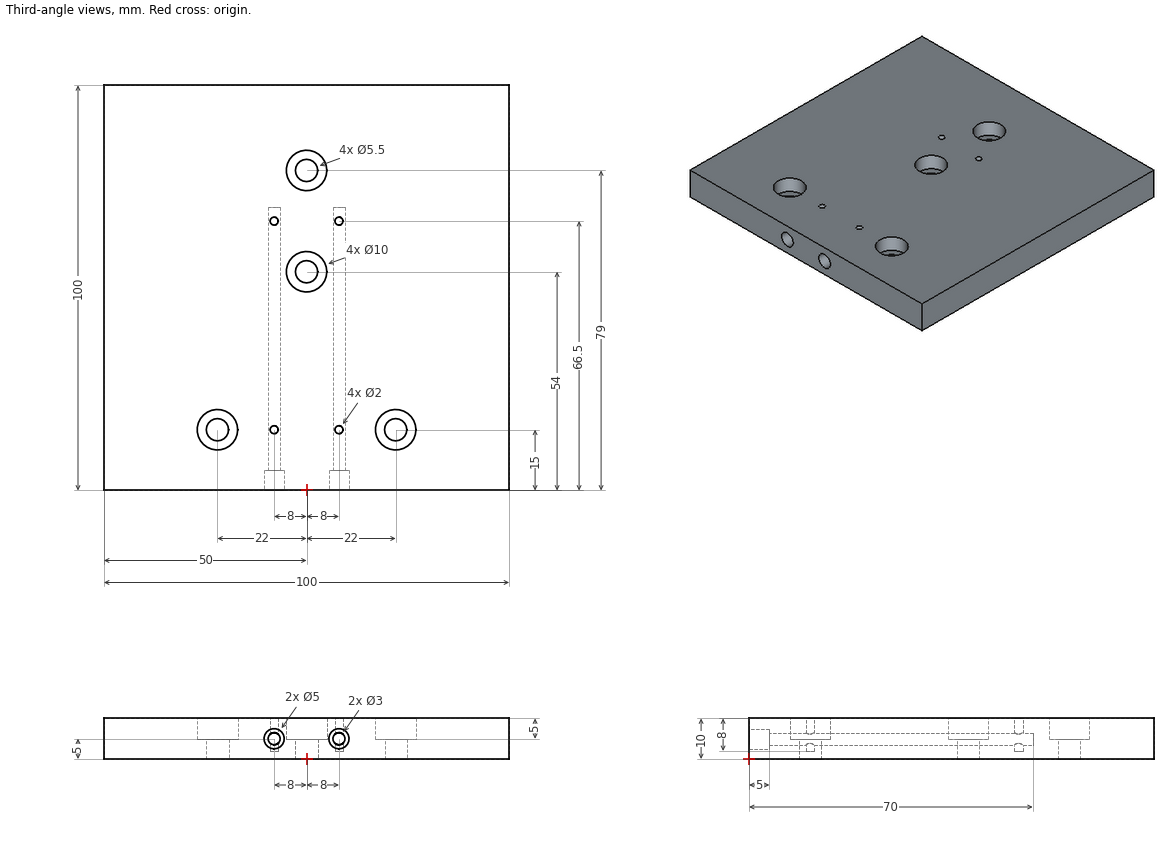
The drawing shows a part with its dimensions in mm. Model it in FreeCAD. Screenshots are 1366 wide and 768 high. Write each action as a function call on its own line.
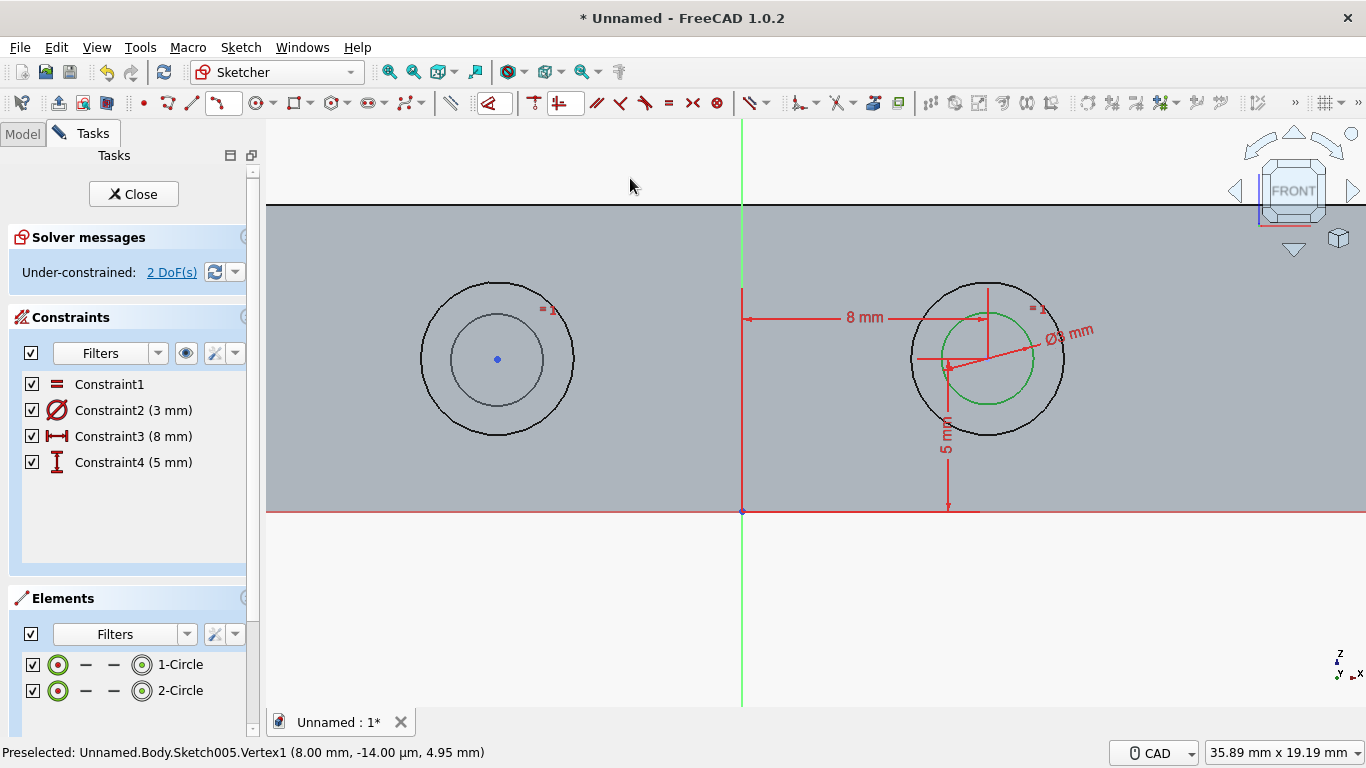
click(497, 360)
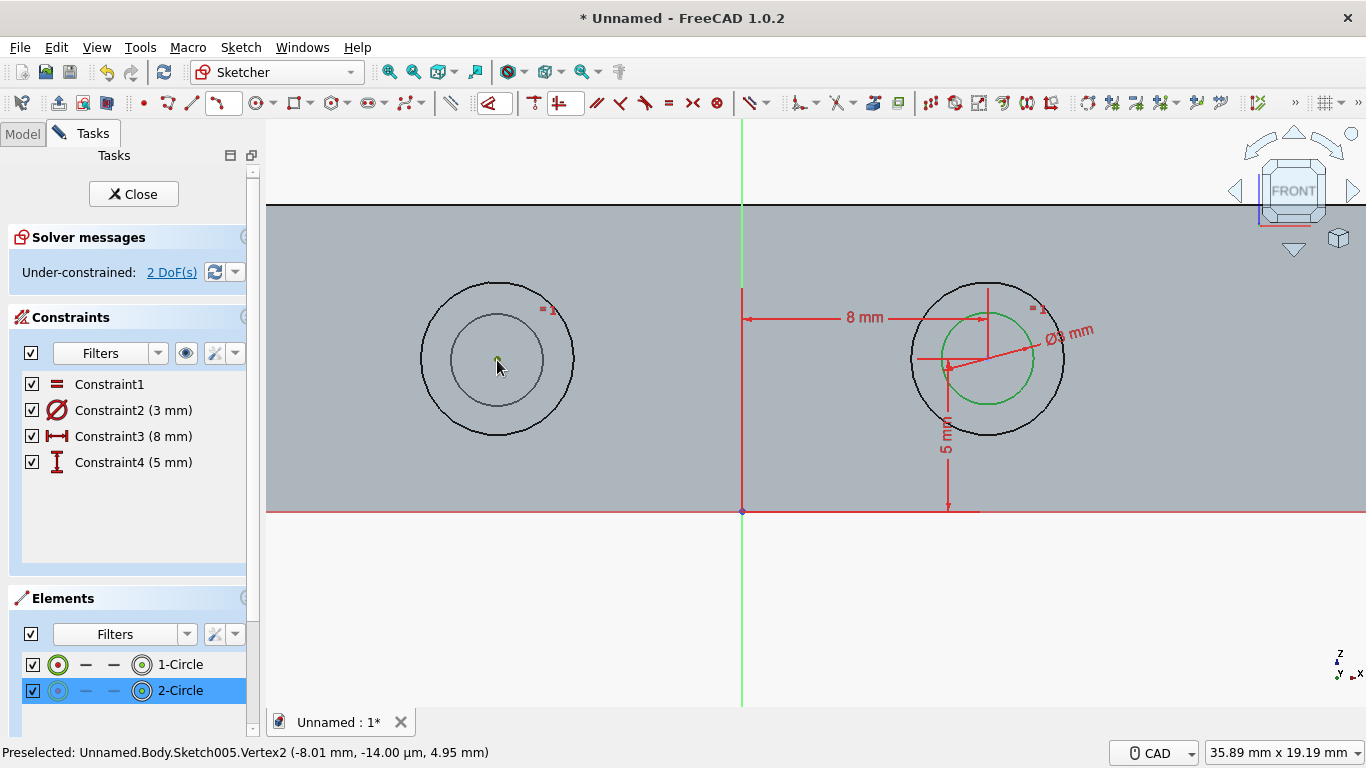
key(l)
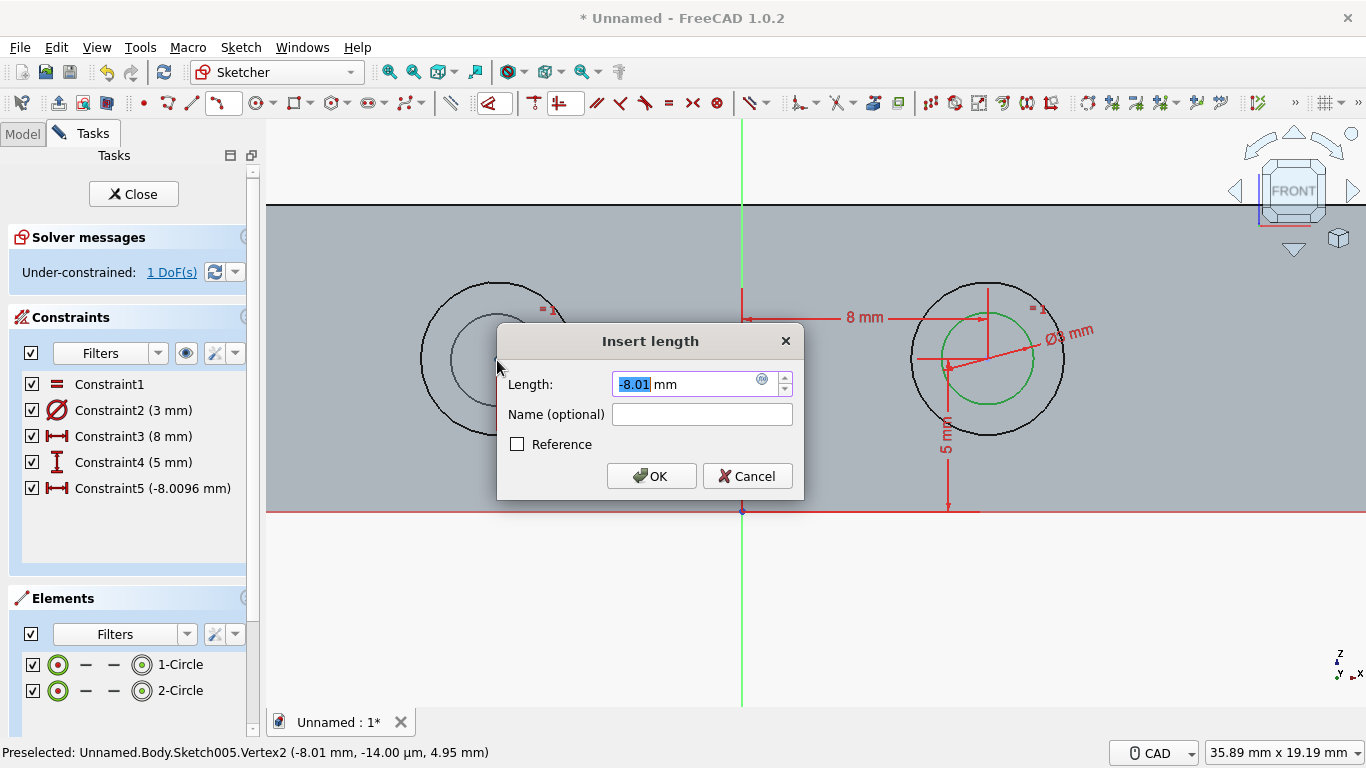
text(-8)
key(Return)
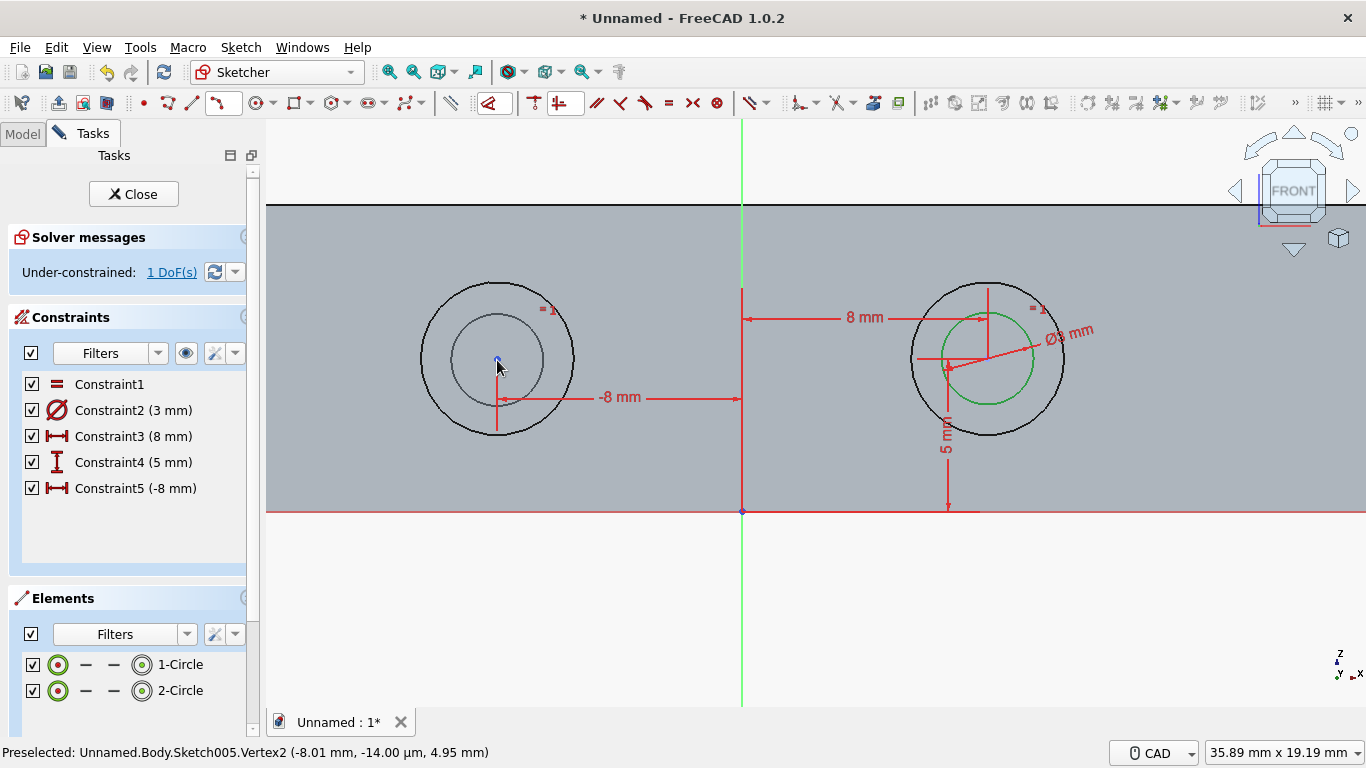
click(497, 360)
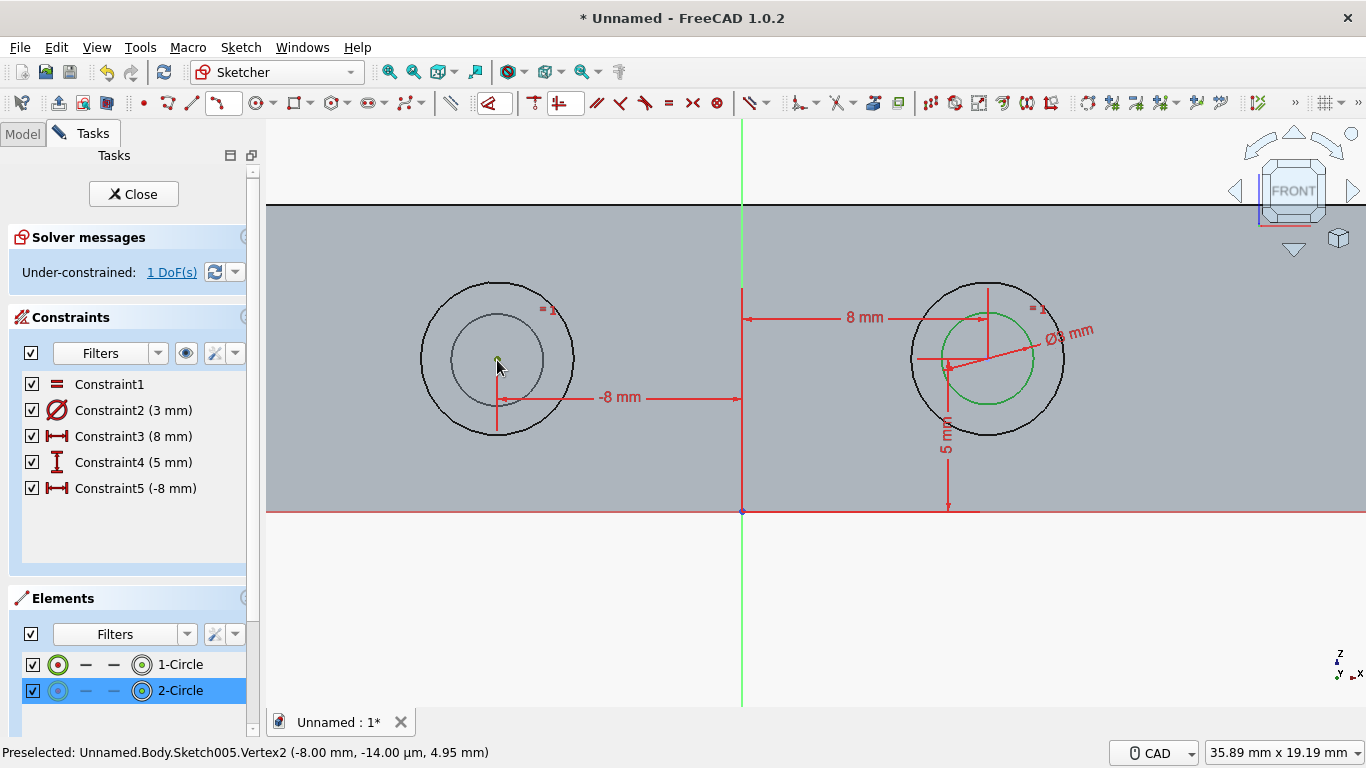
key(i)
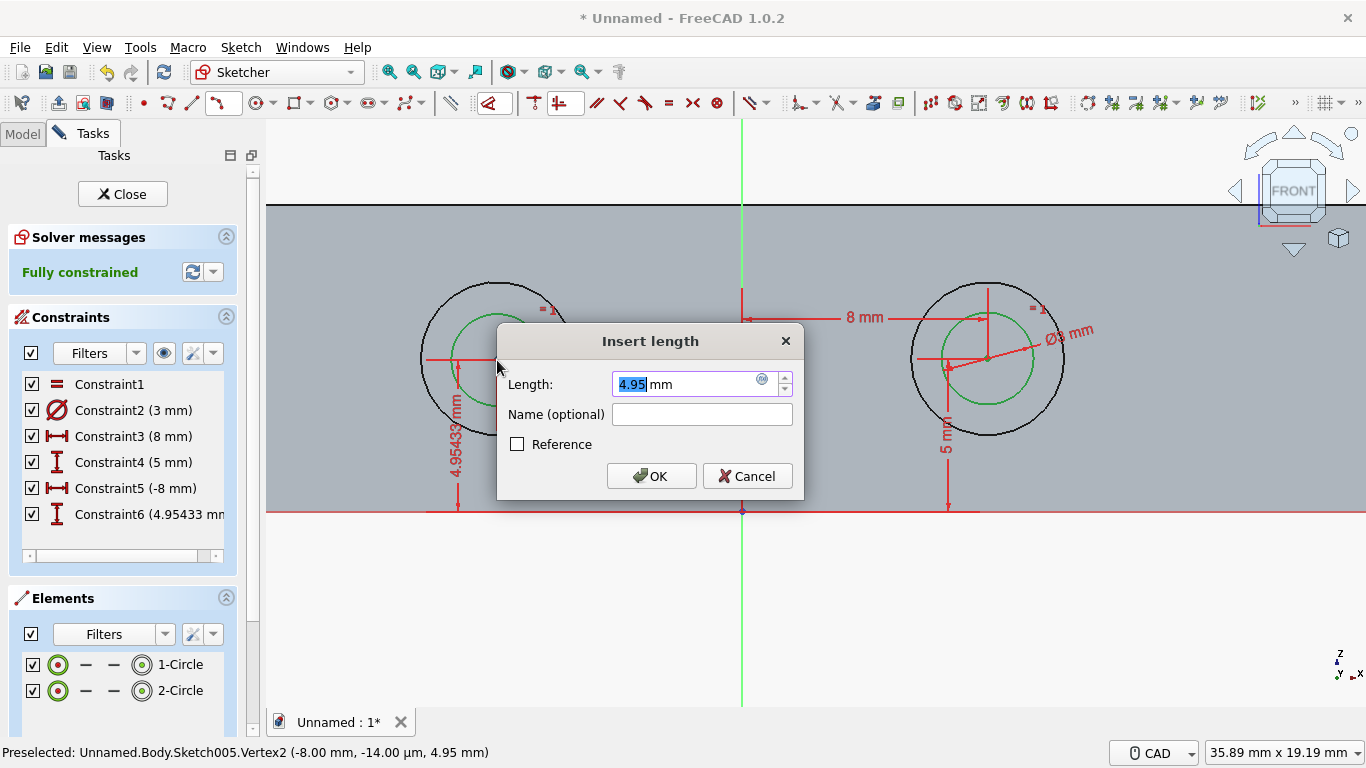
text(5)
key(Return)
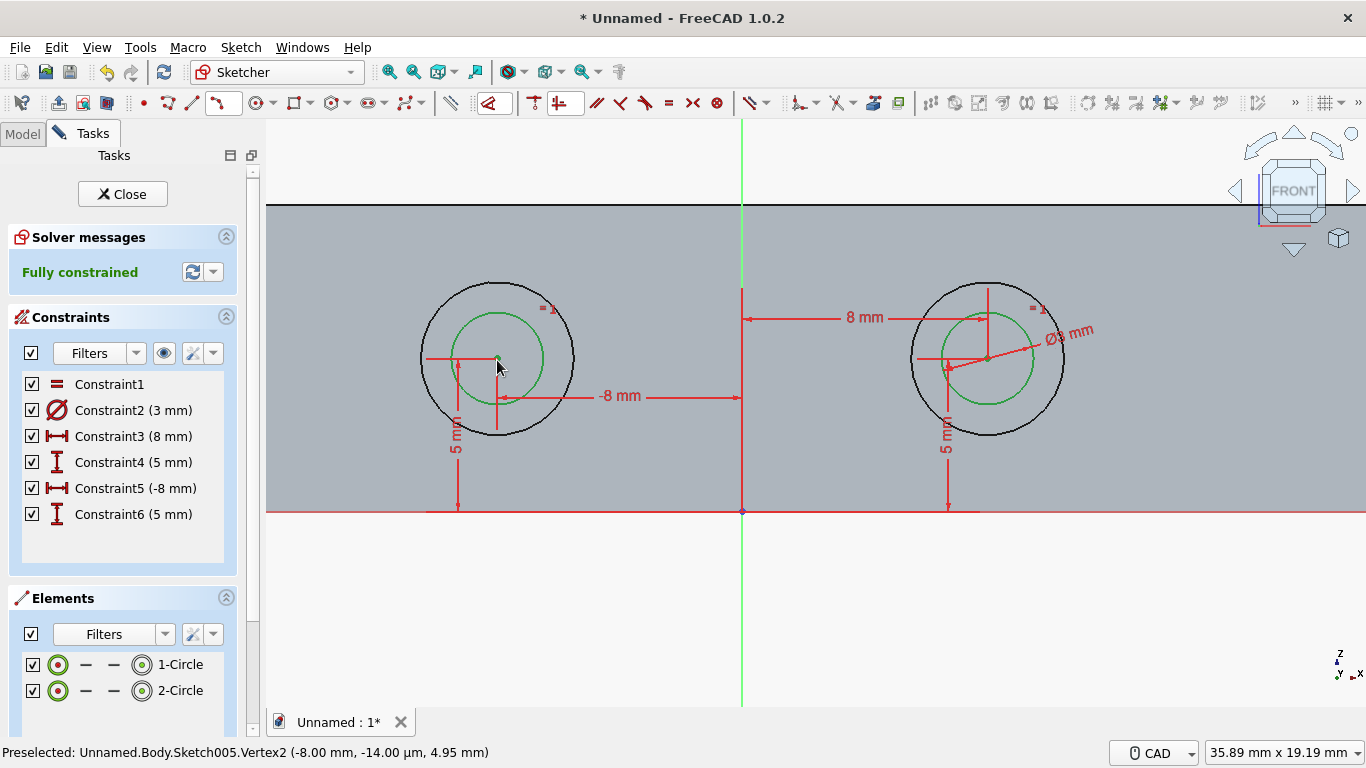
click(123, 194)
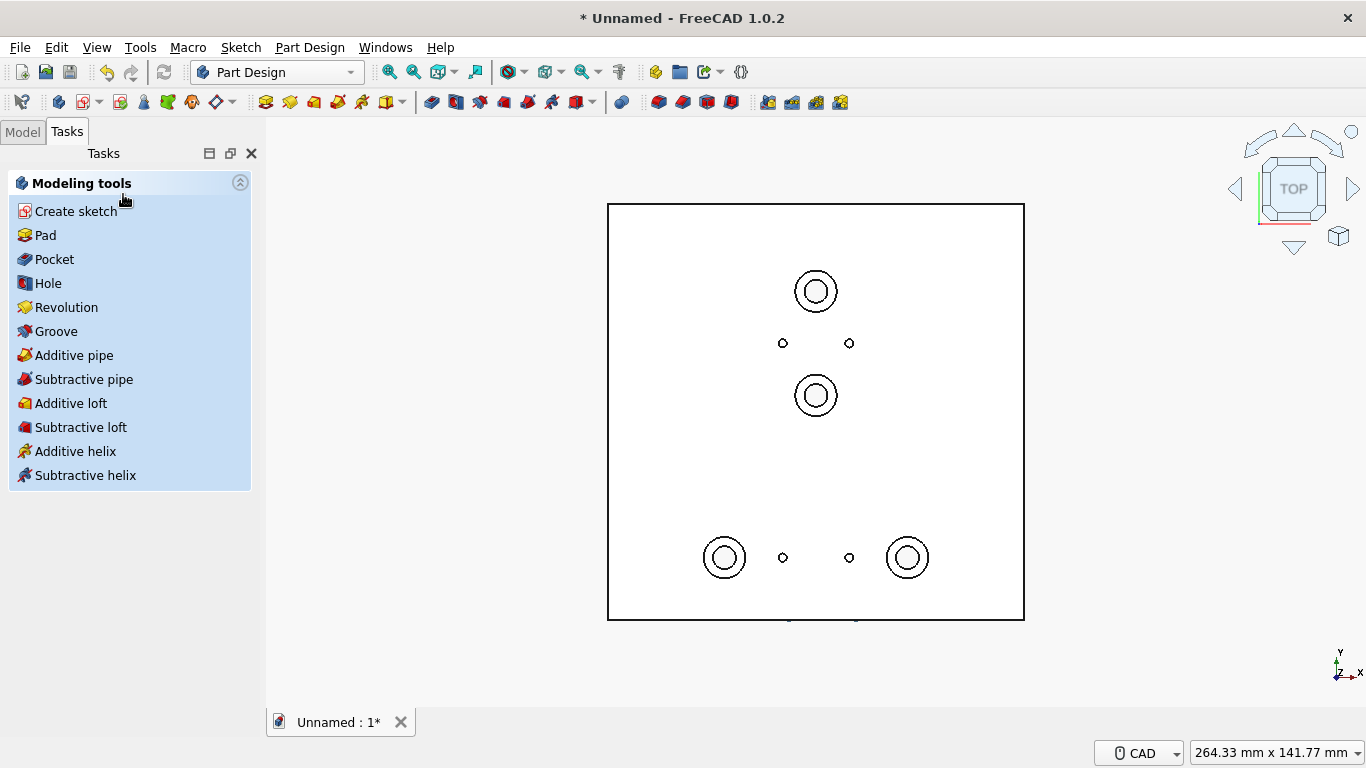
click(432, 102)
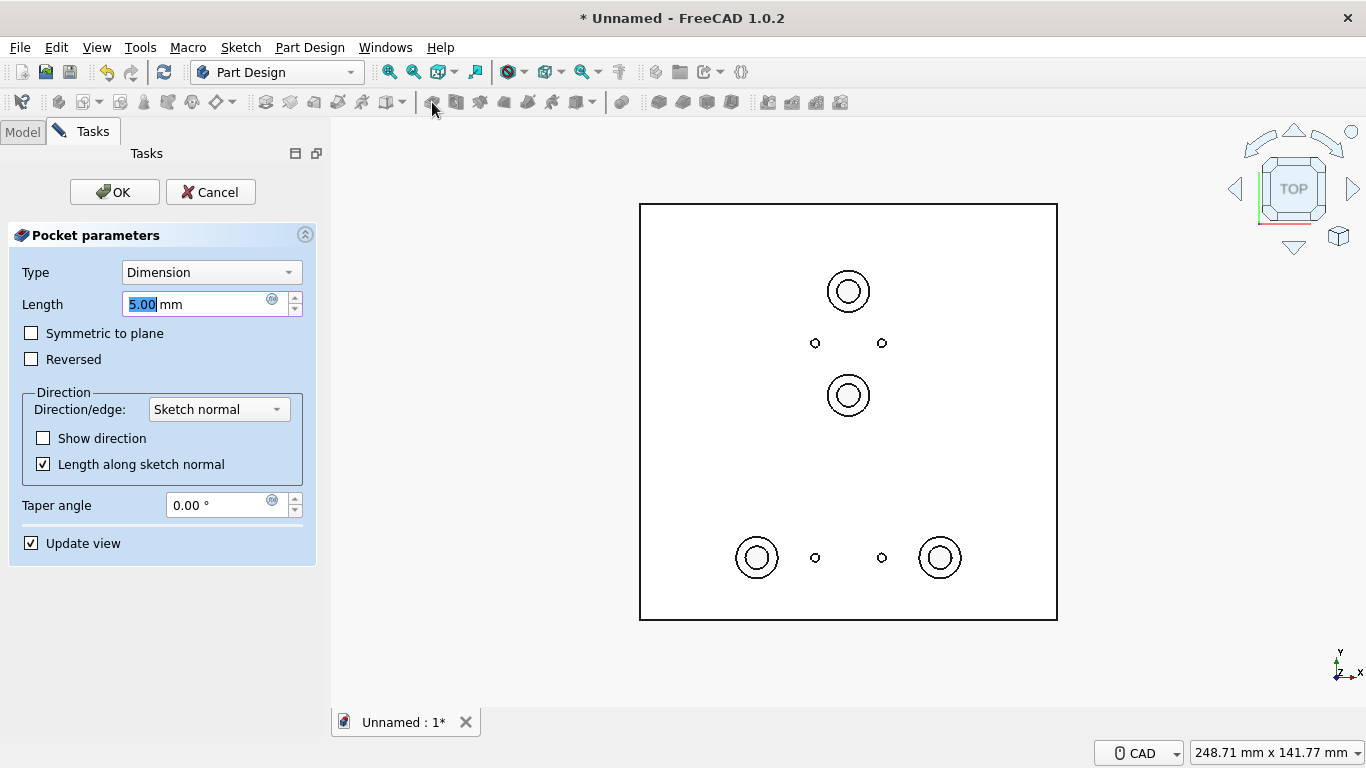
text(70)
key(Tab)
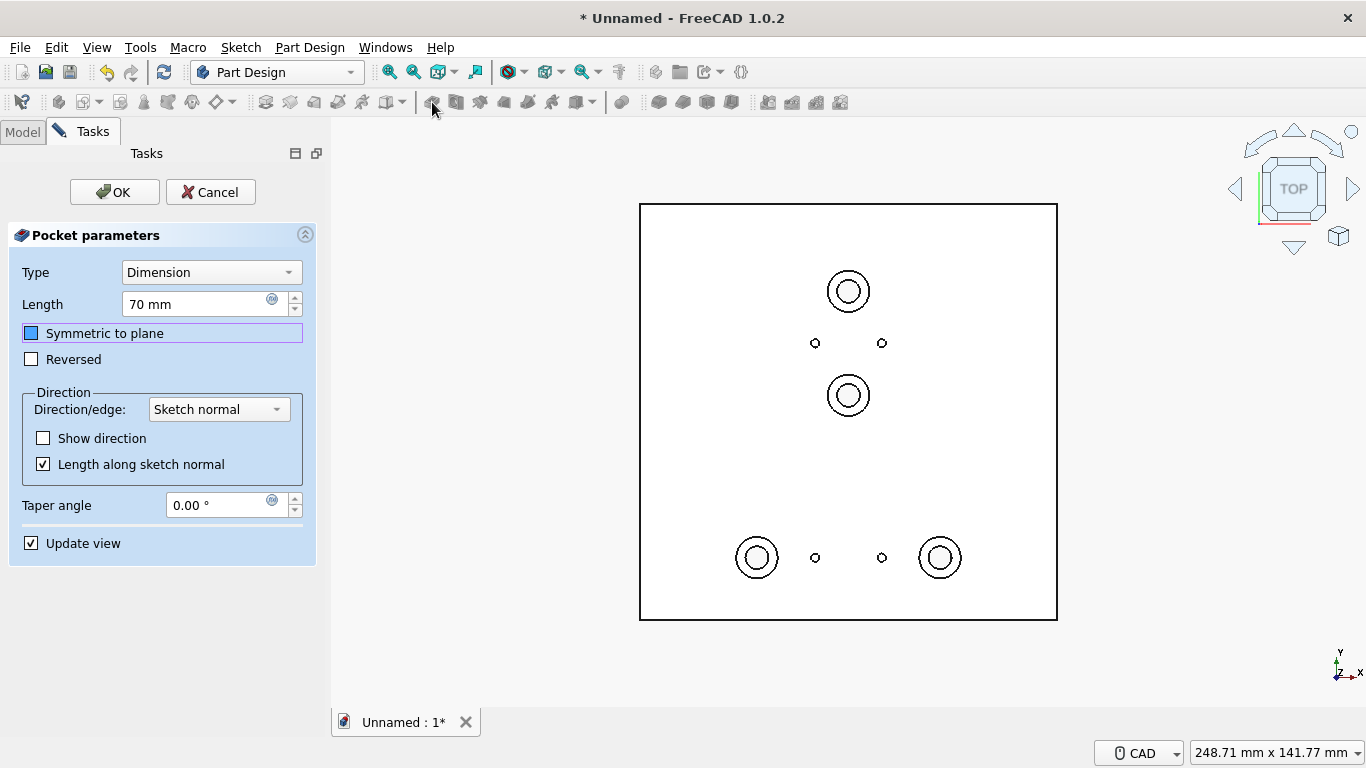
click(115, 192)